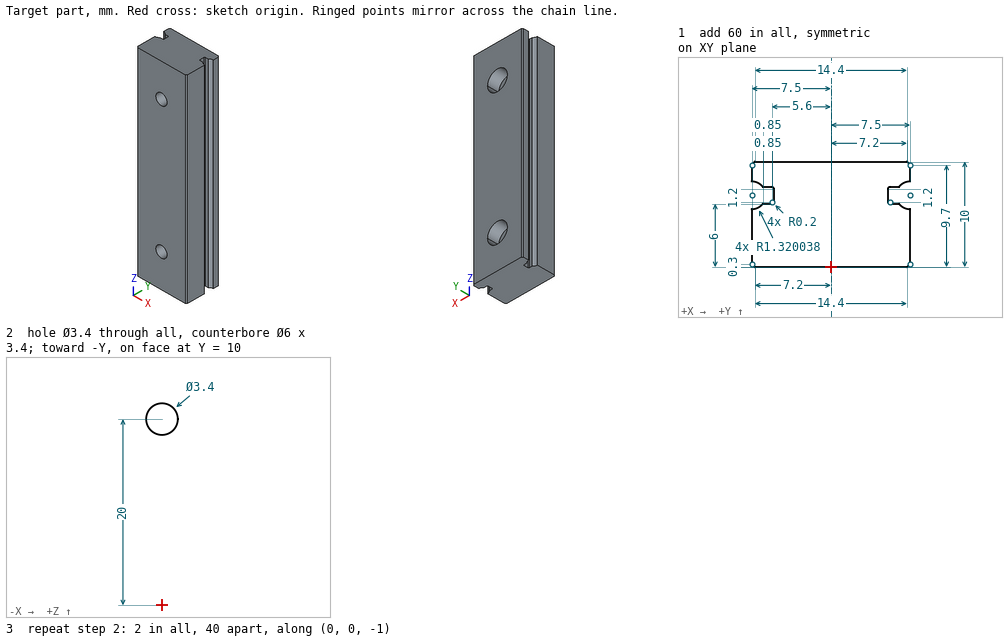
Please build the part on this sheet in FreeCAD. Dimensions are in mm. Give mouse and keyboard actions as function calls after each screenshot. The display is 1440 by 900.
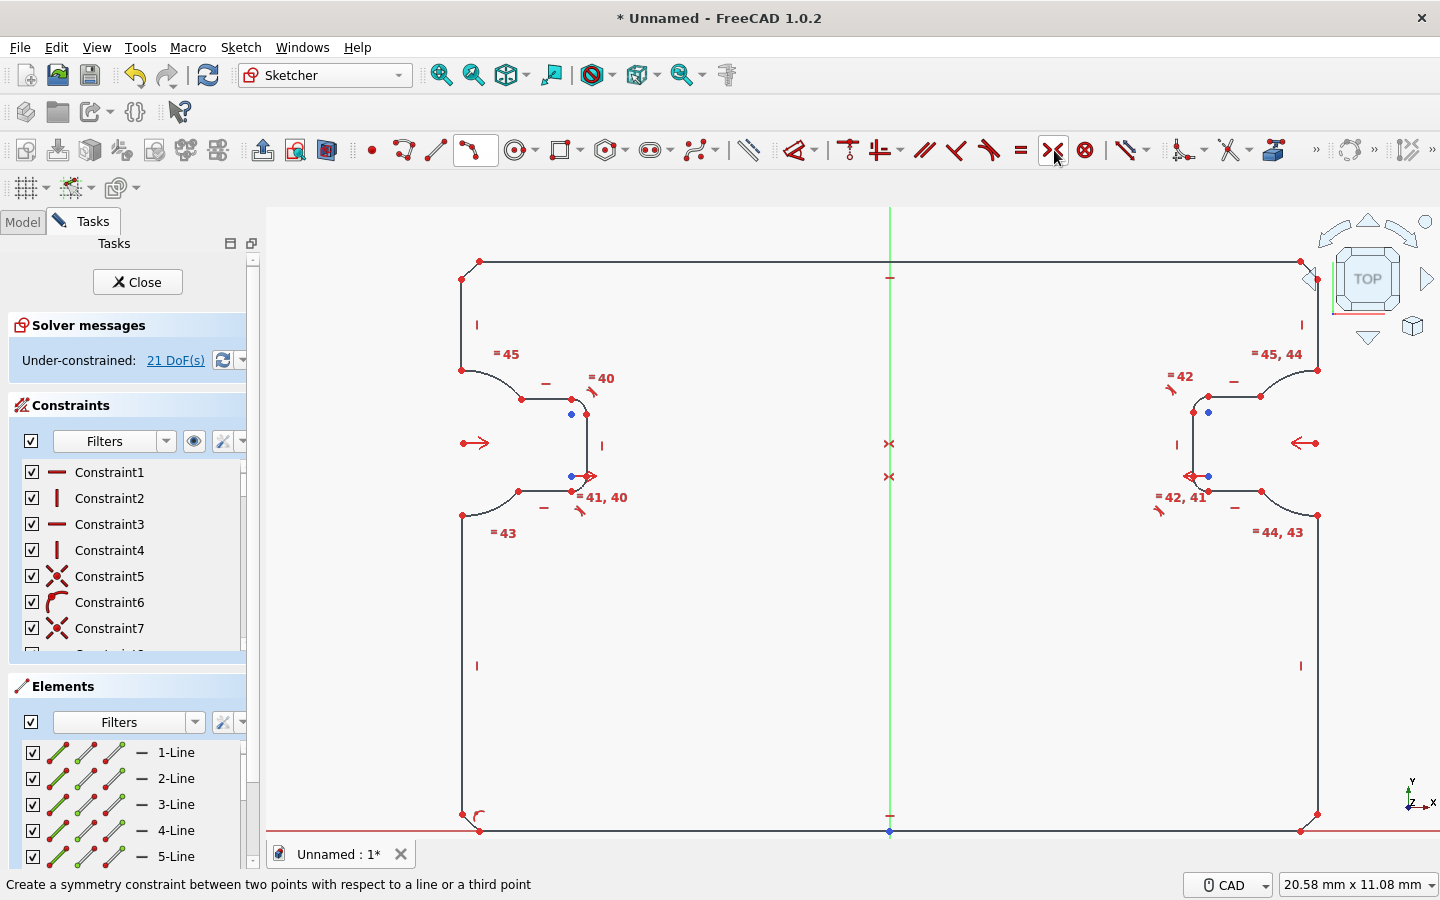
scroll(570, 477, down, 2)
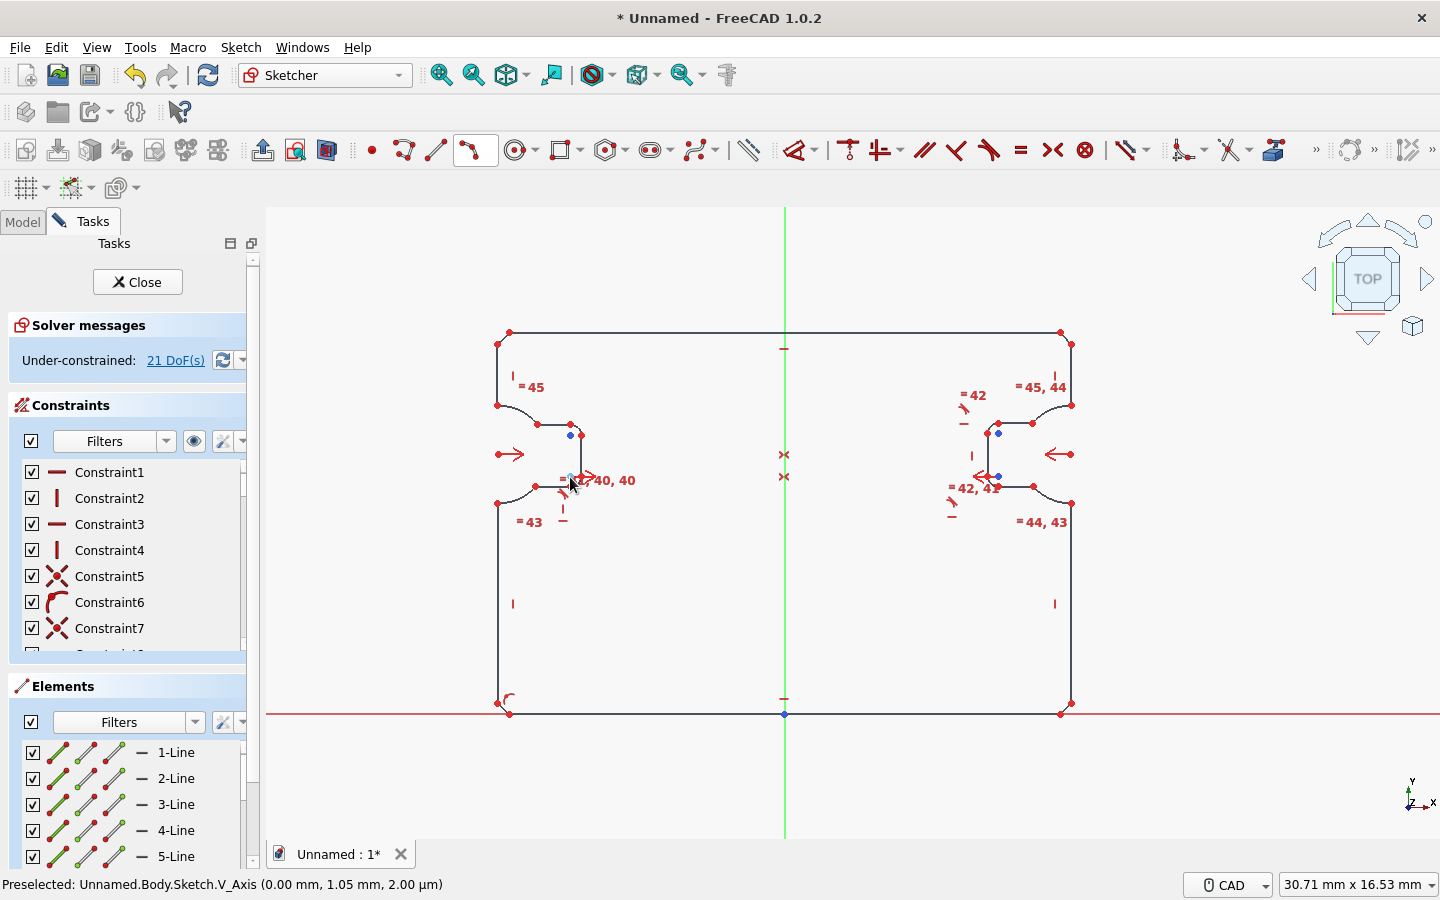
click(498, 703)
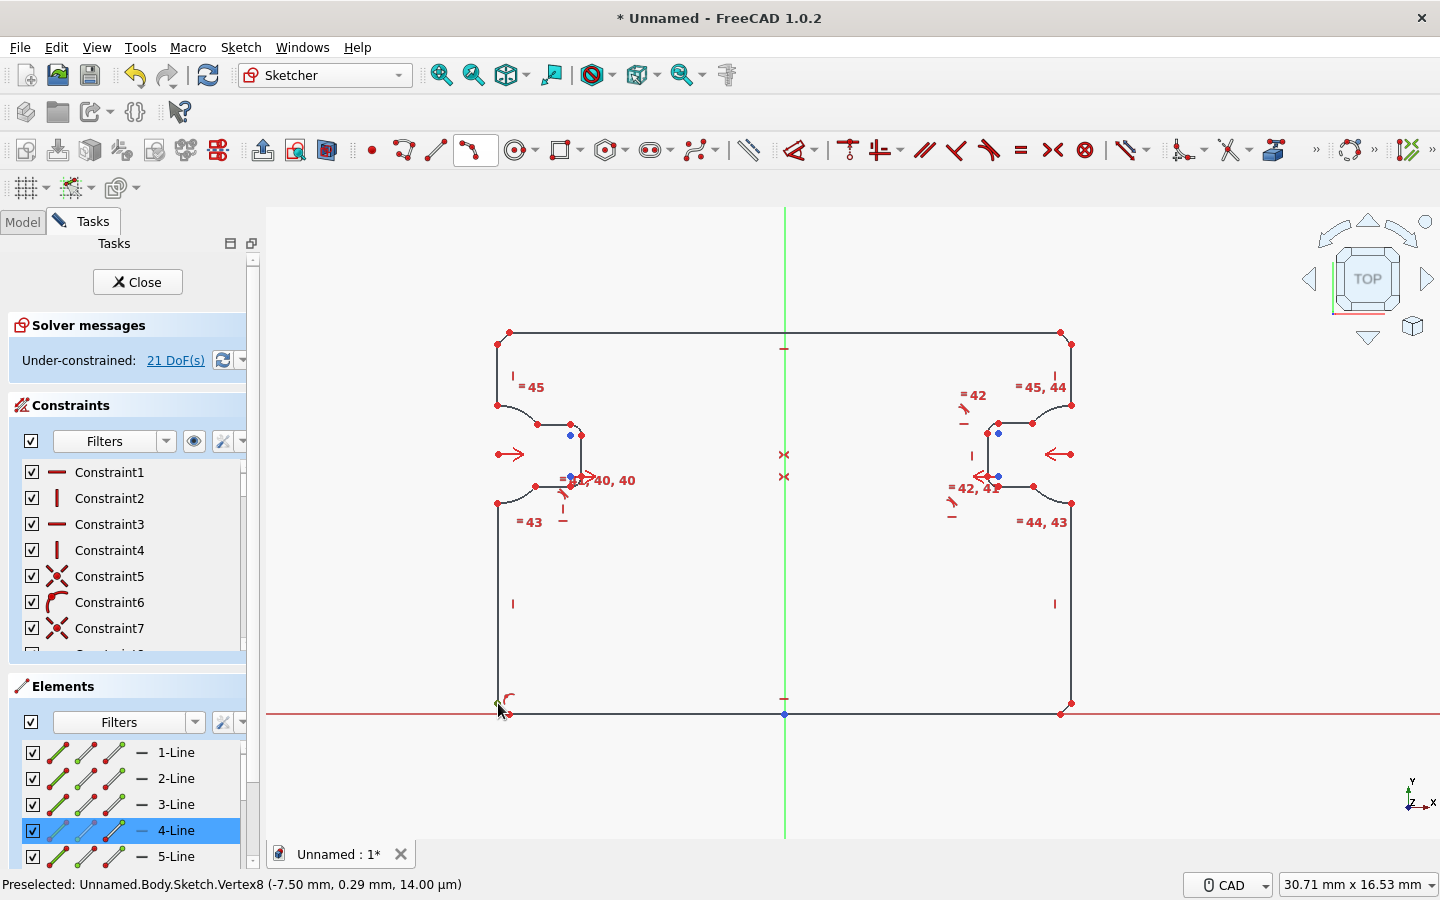
click(1071, 703)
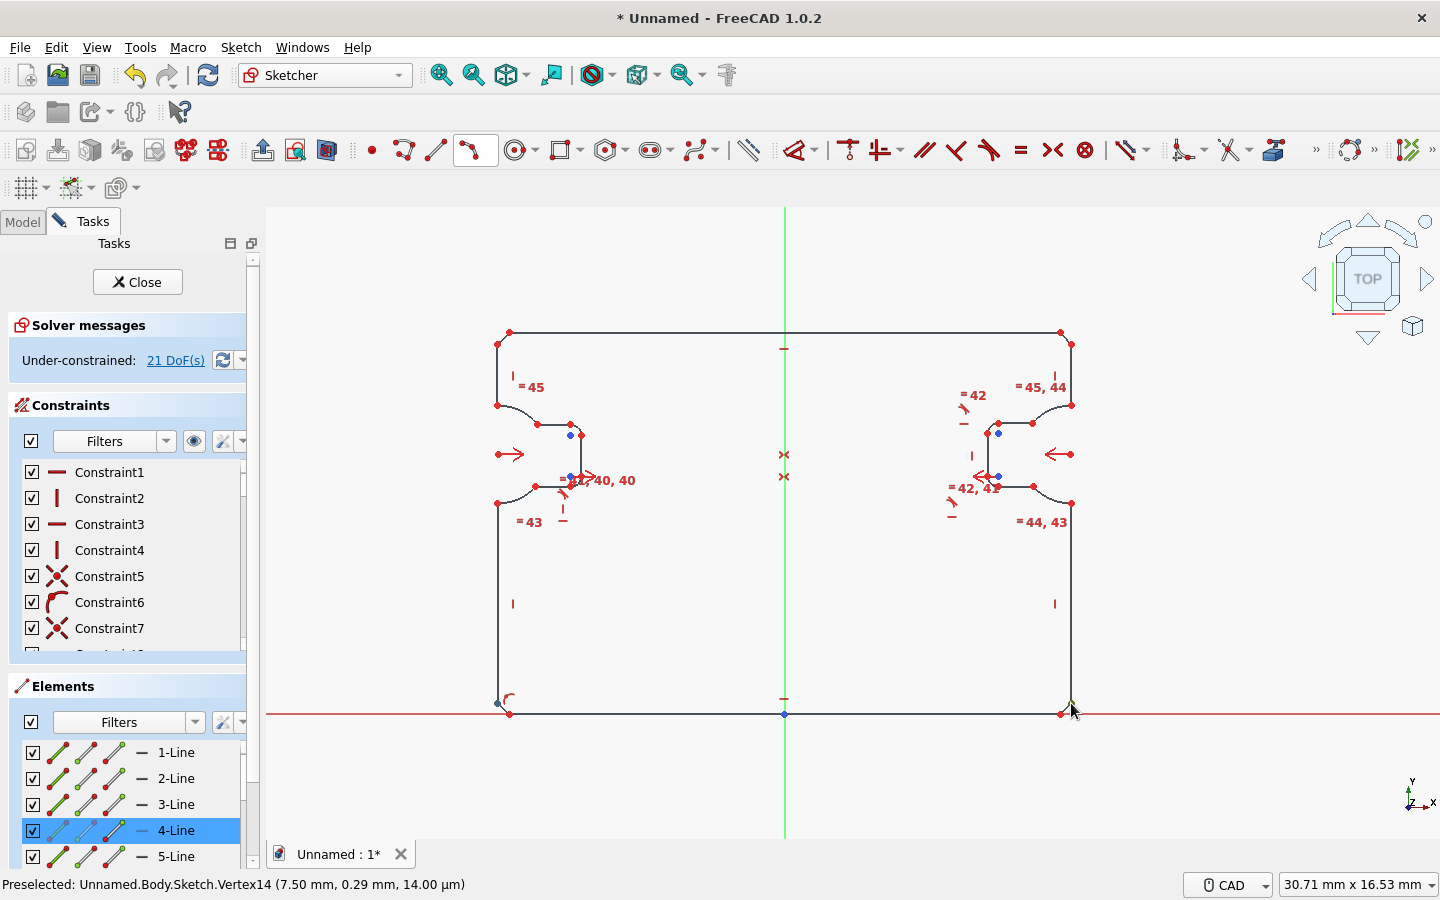
click(785, 770)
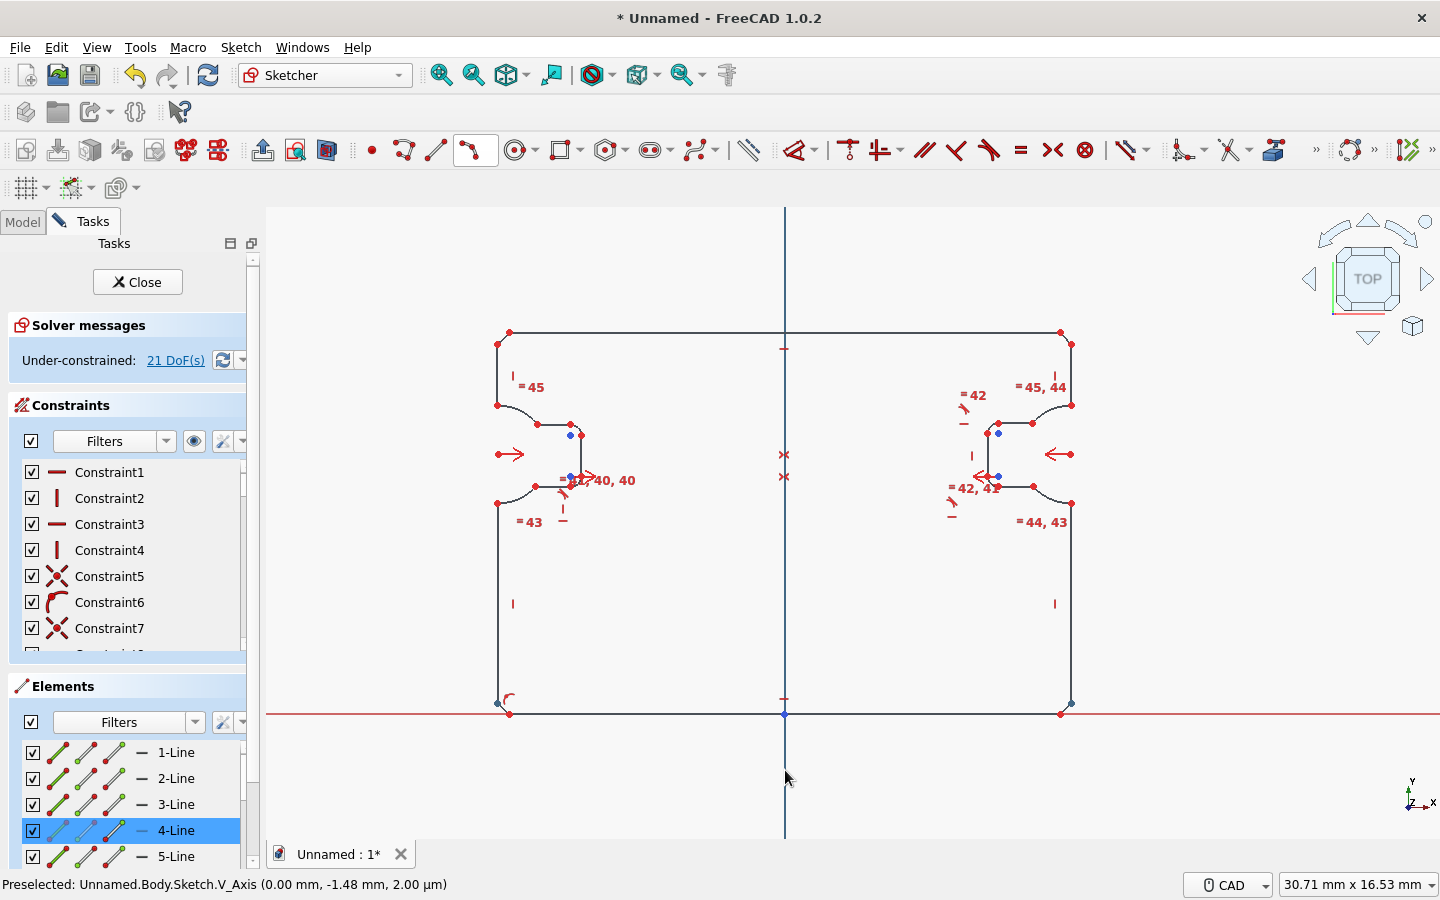
click(1054, 150)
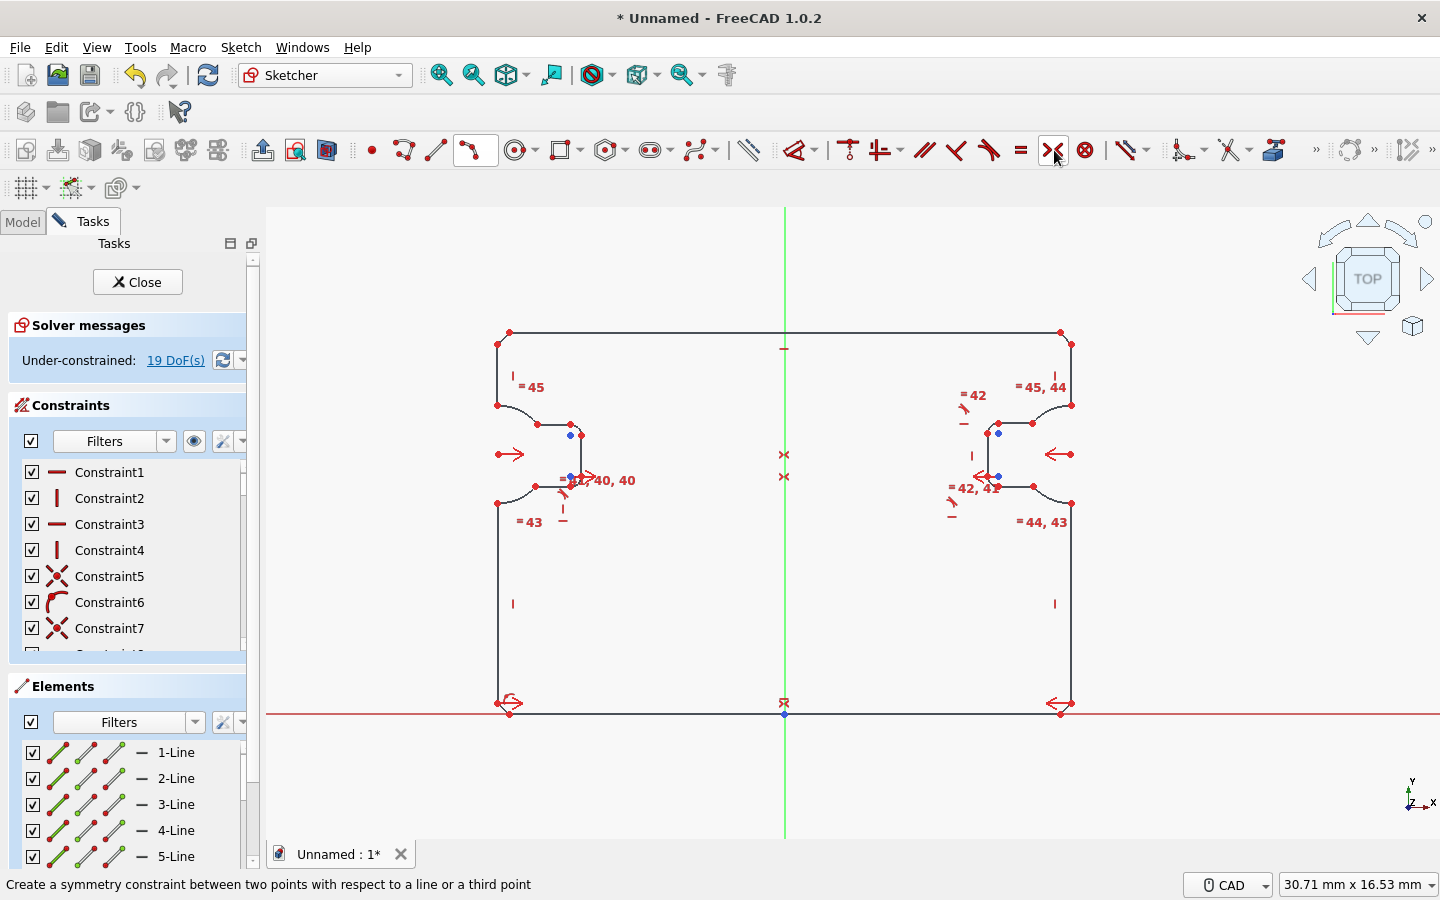
click(1071, 345)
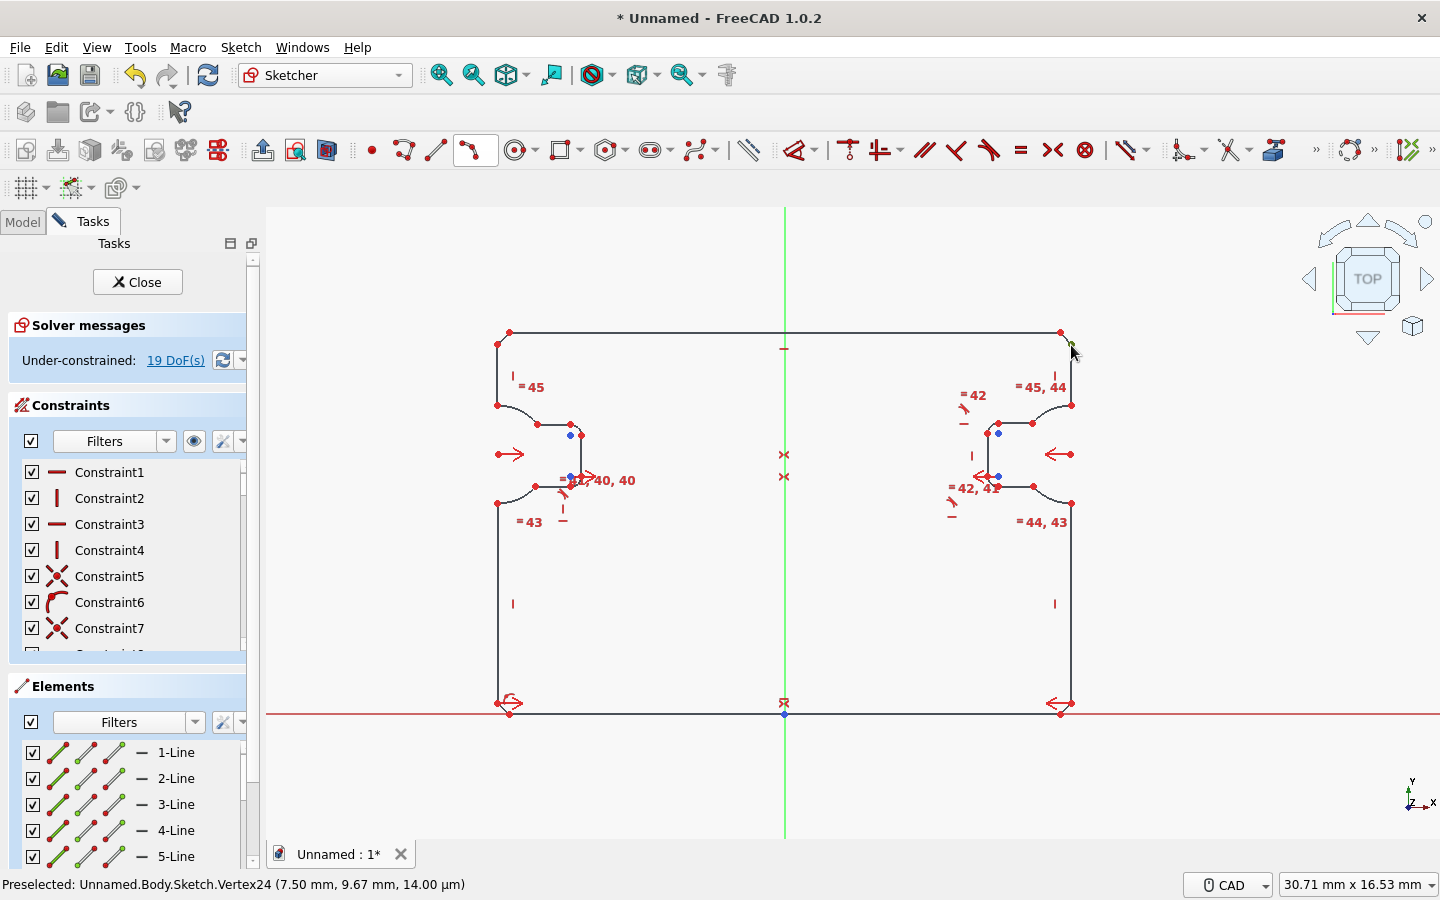
click(497, 345)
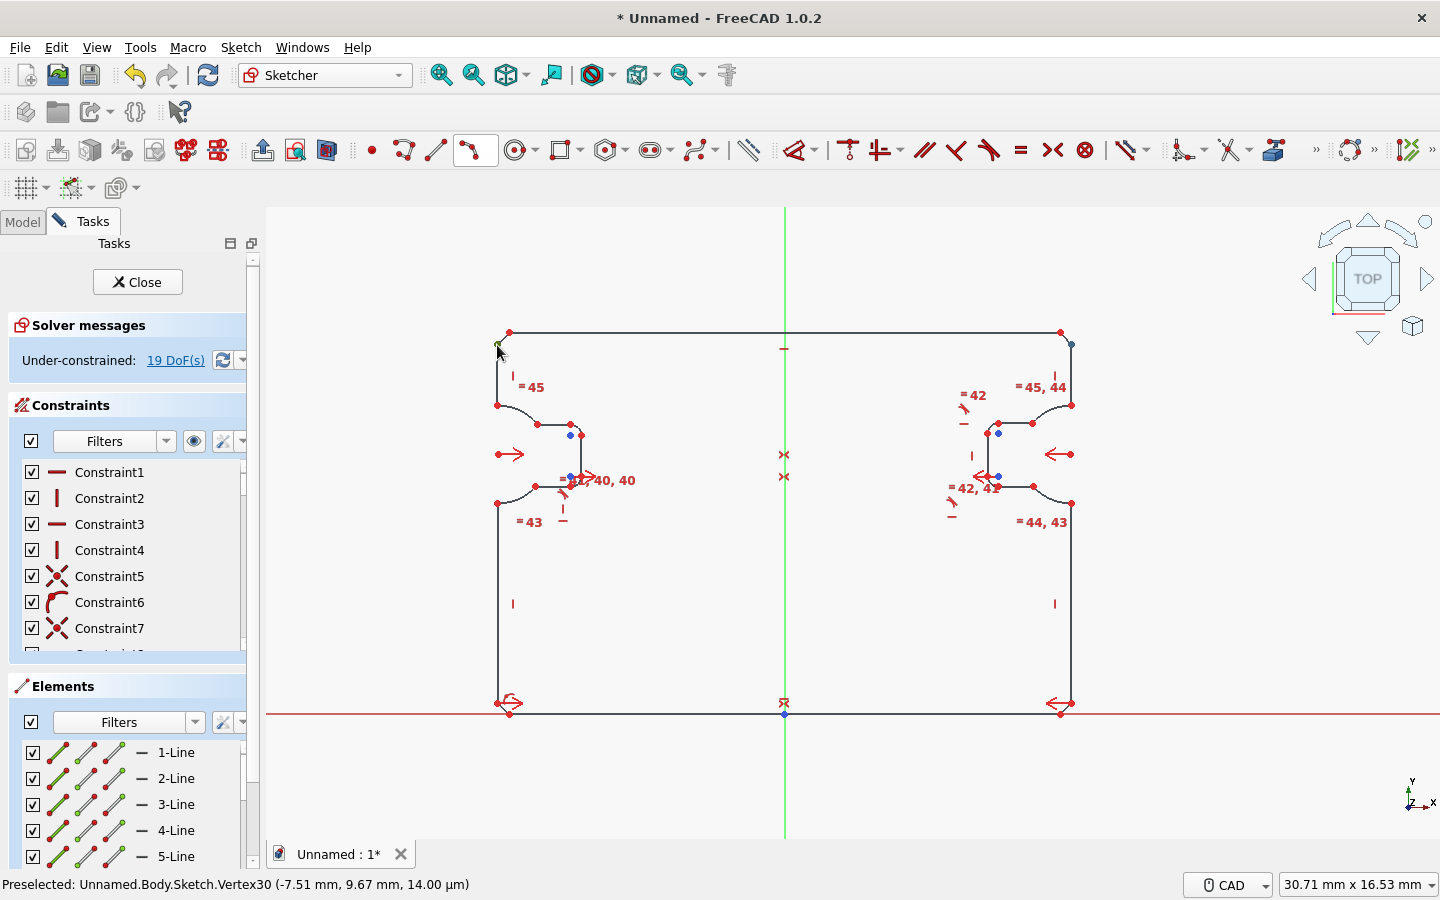
click(785, 770)